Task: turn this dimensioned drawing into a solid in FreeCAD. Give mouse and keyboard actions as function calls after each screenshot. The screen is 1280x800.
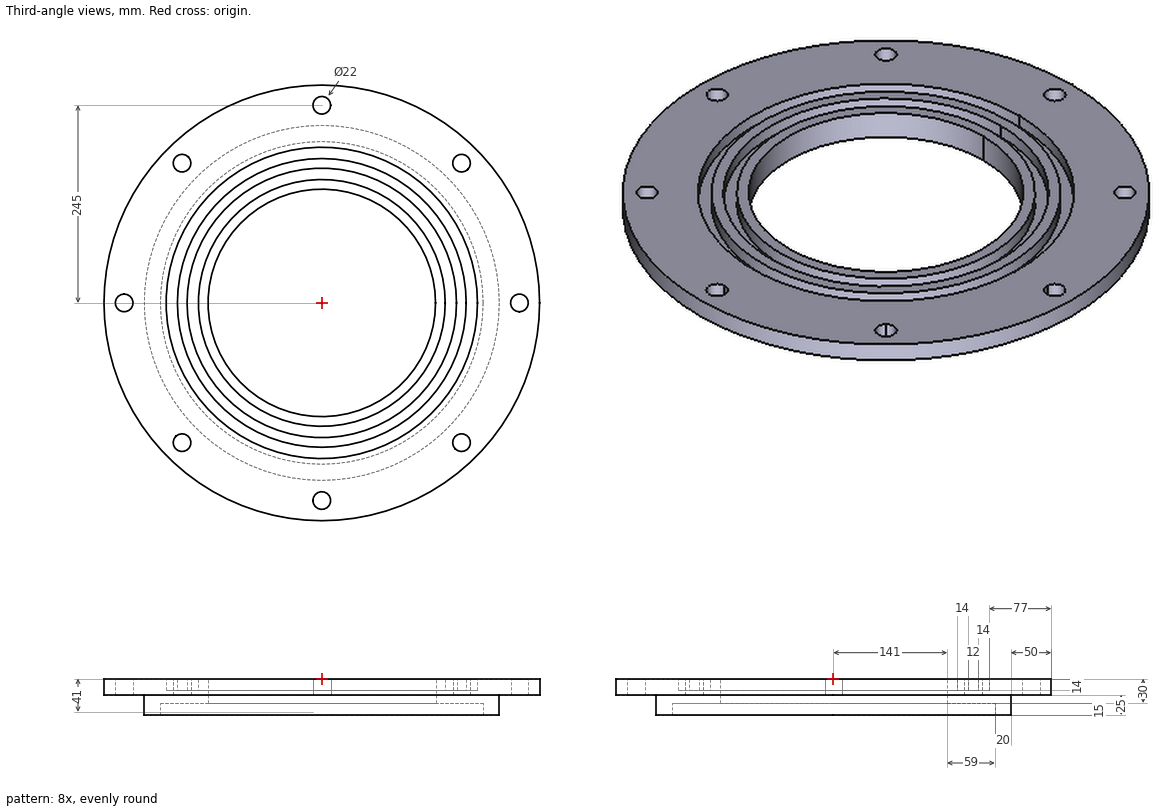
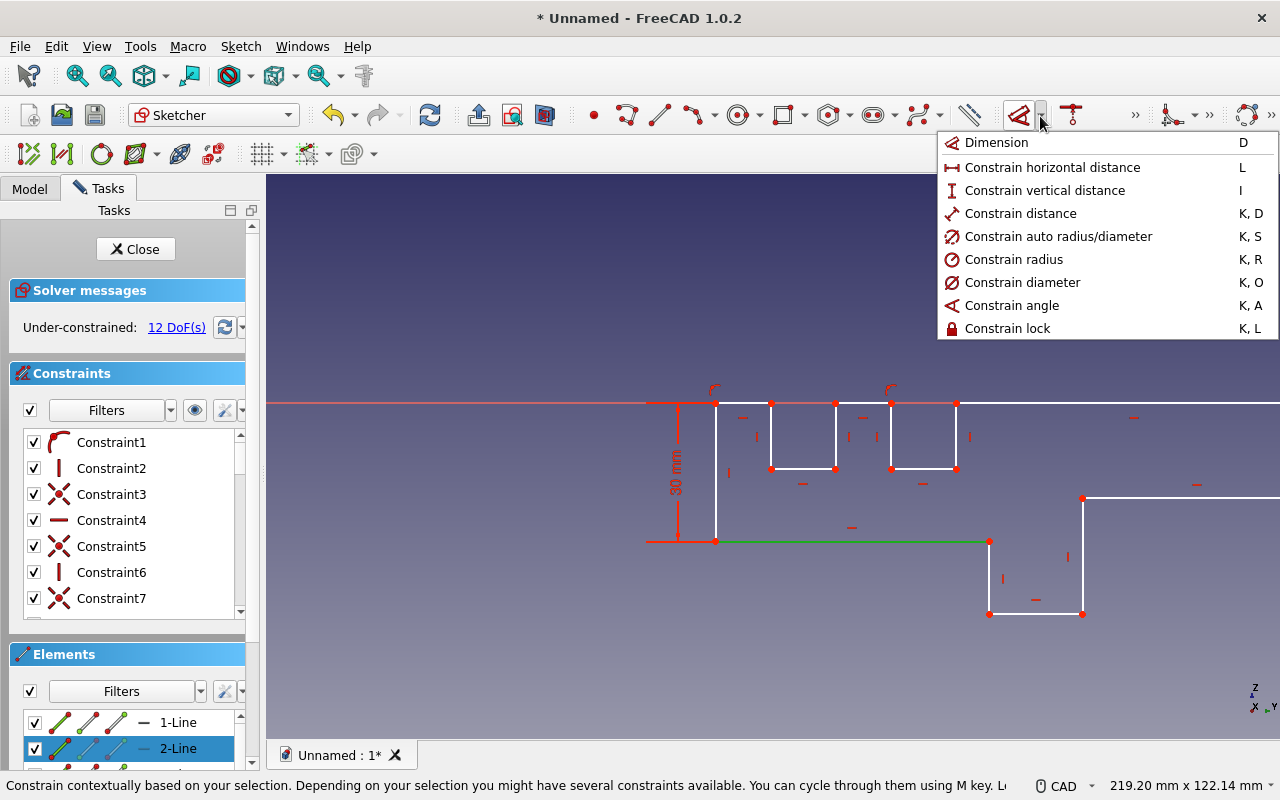
click(1108, 168)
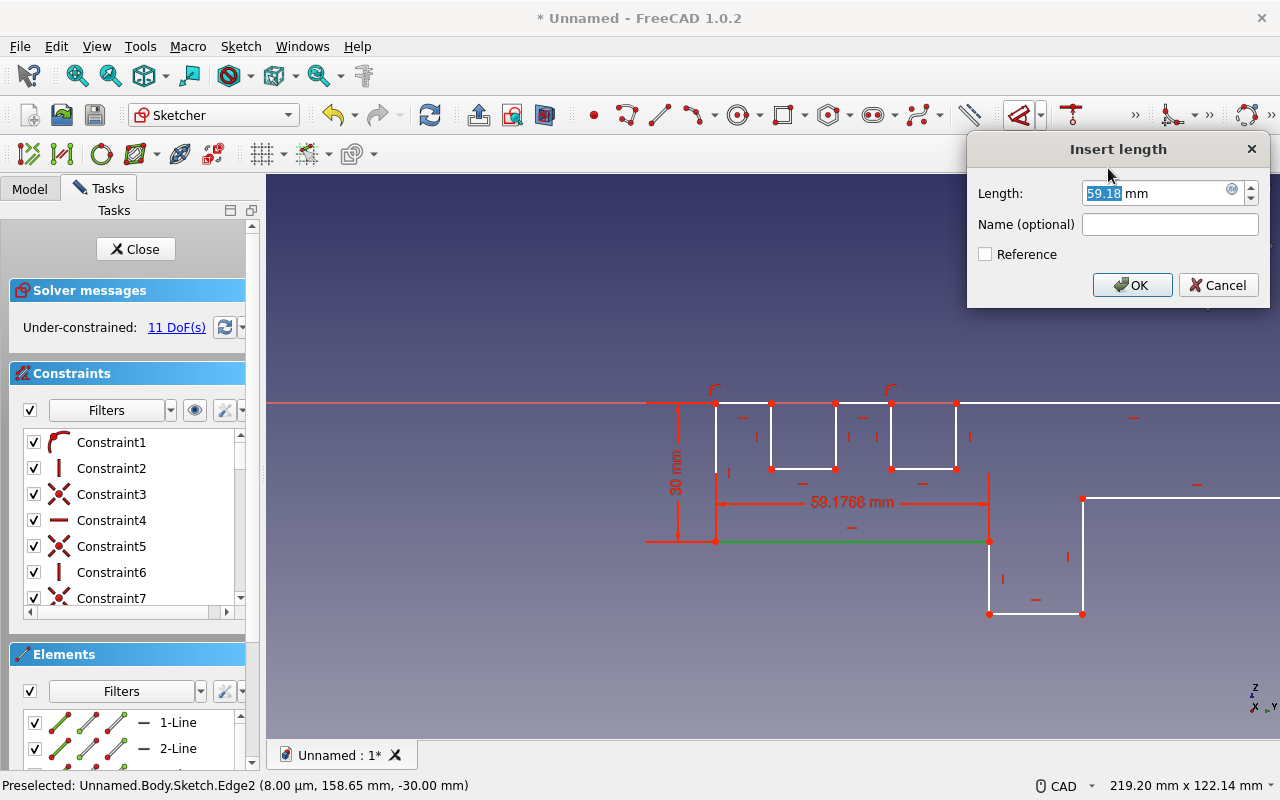
text(59)
key(Return)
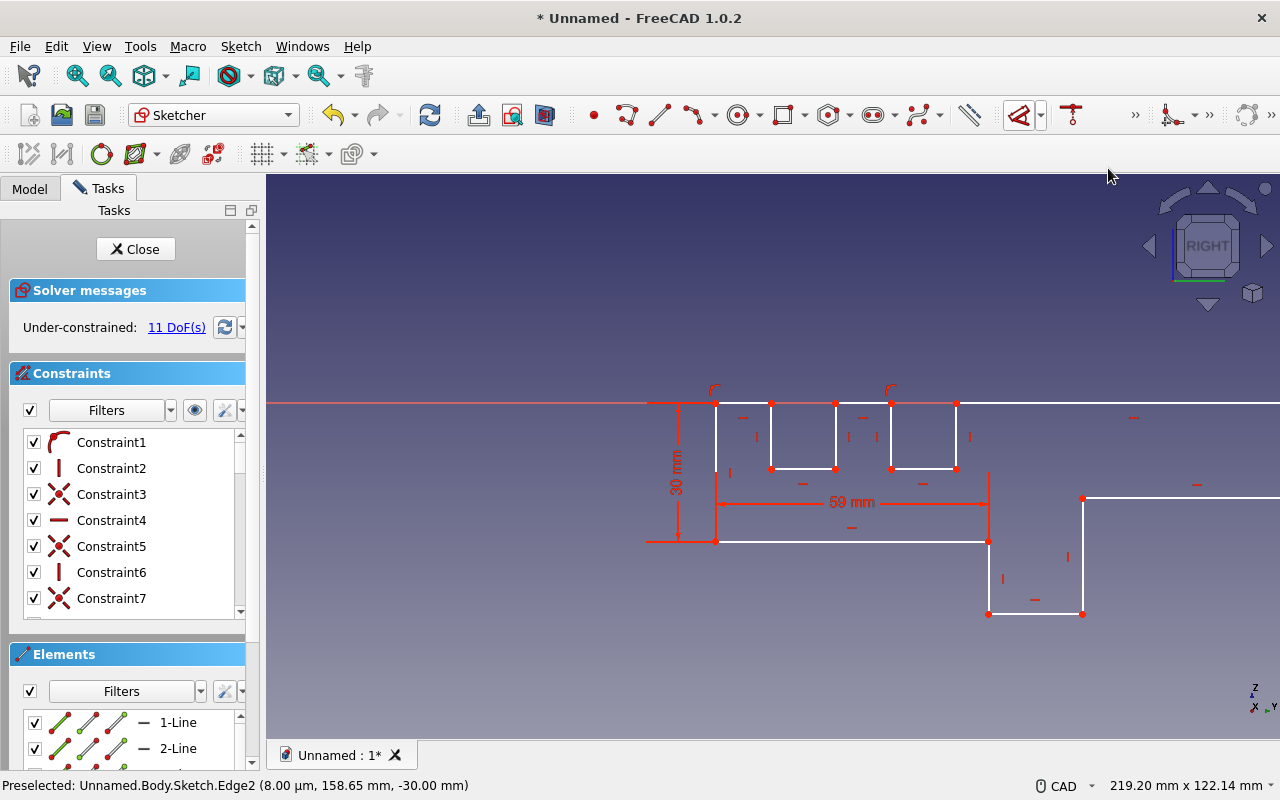
click(989, 564)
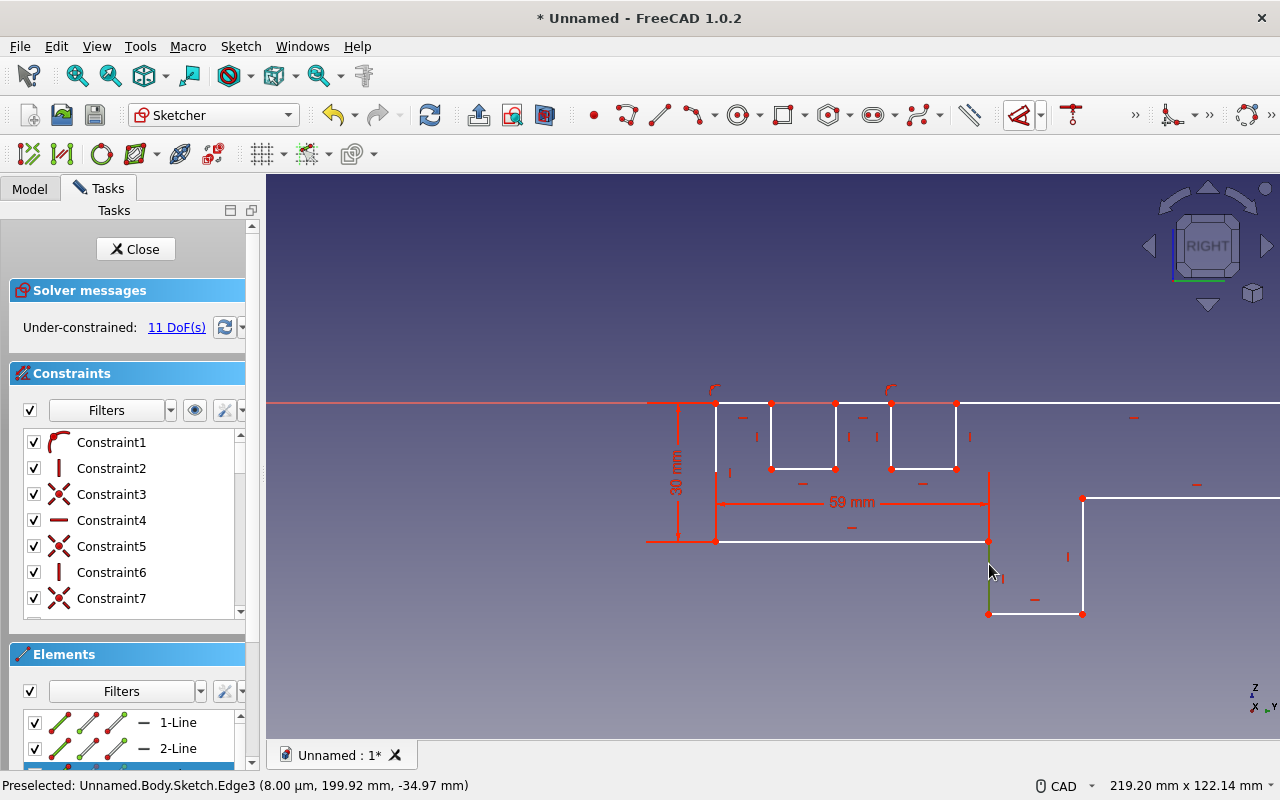
key(i)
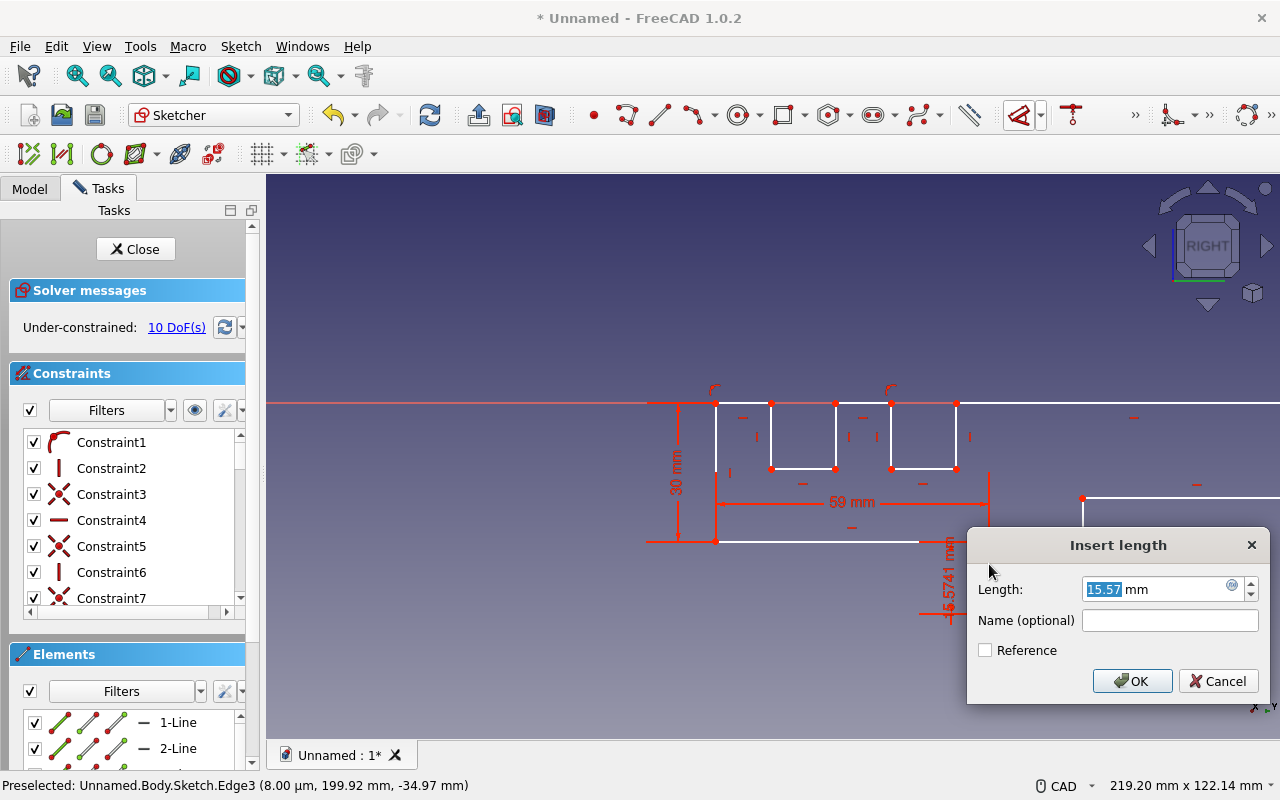
text(15)
key(Return)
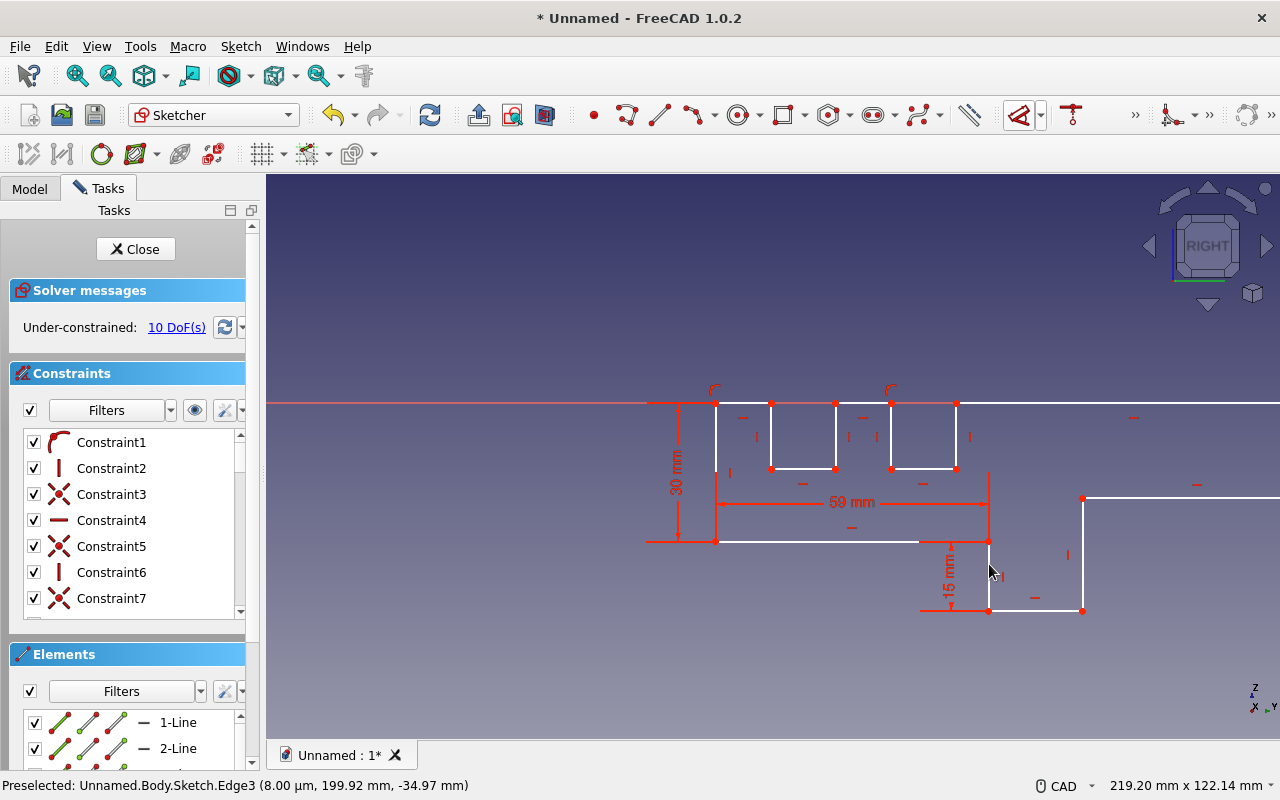
click(1017, 611)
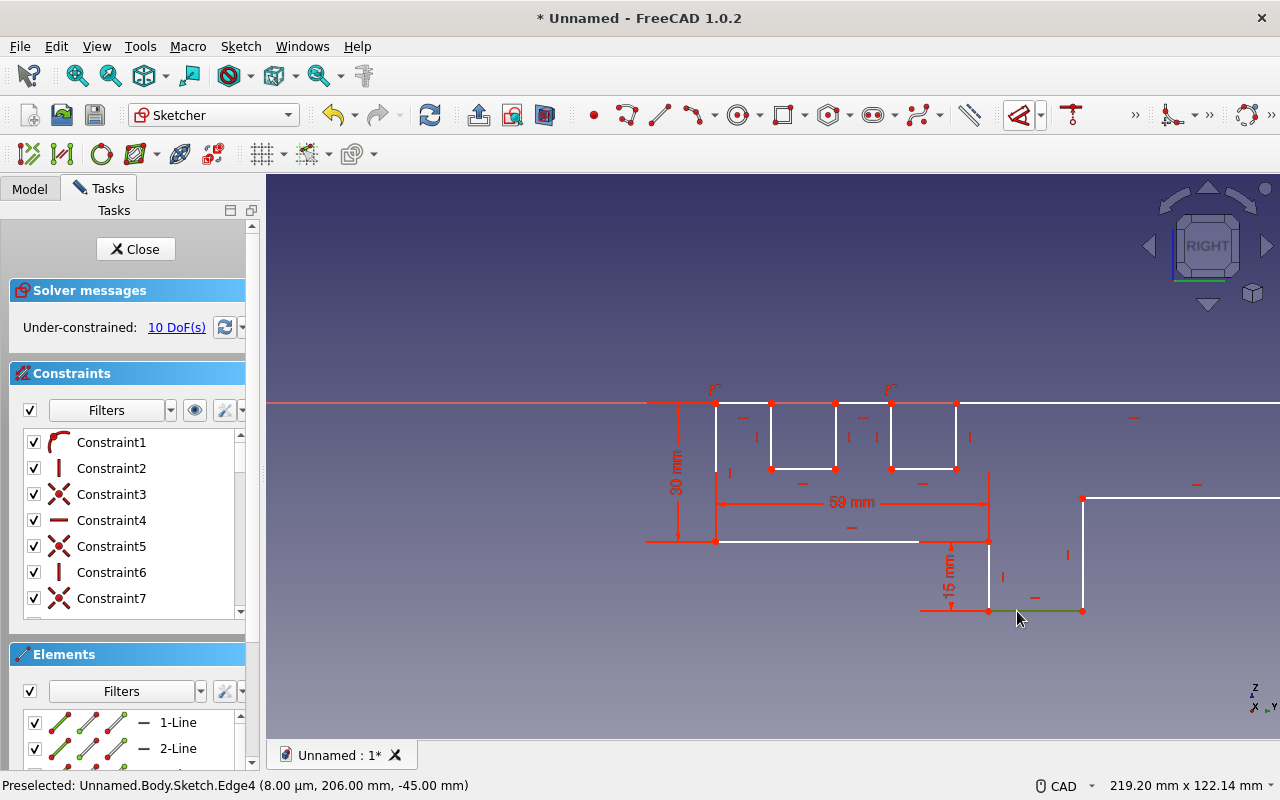
key(l)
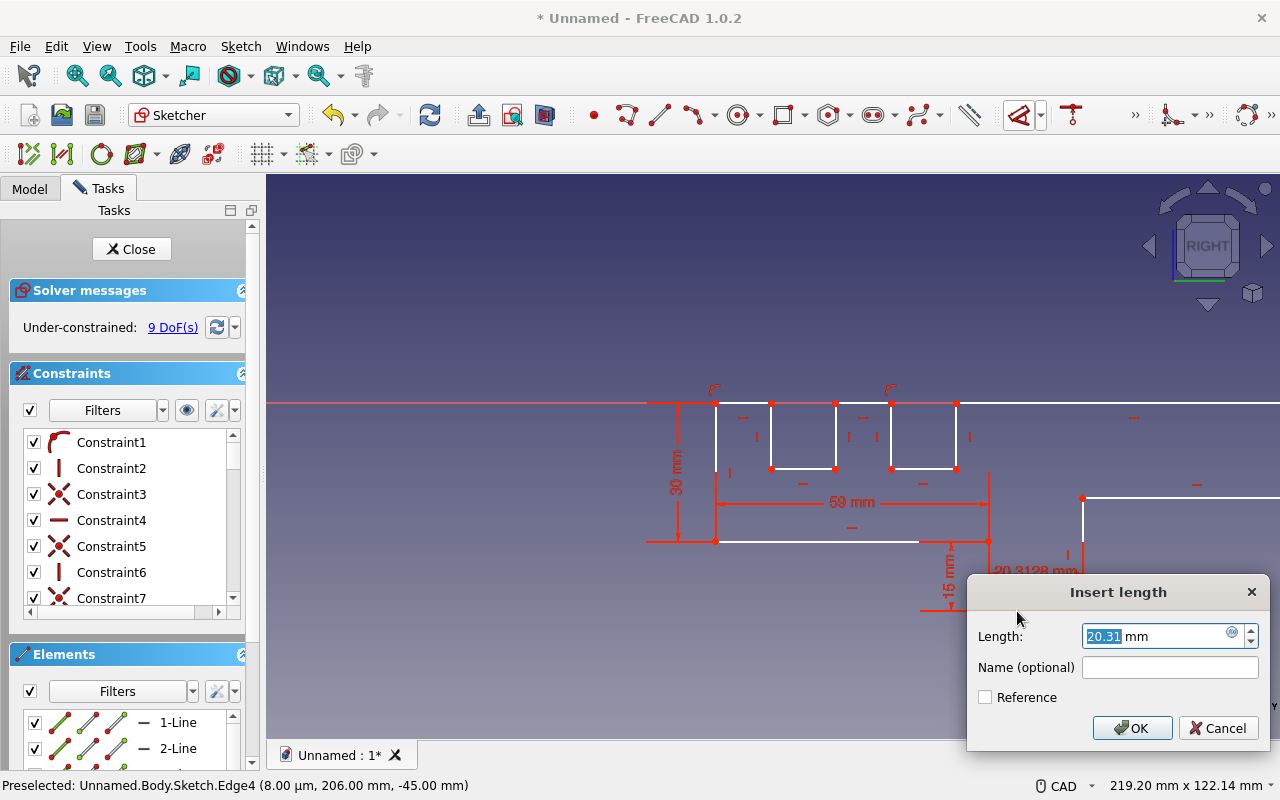
text(20)
key(Return)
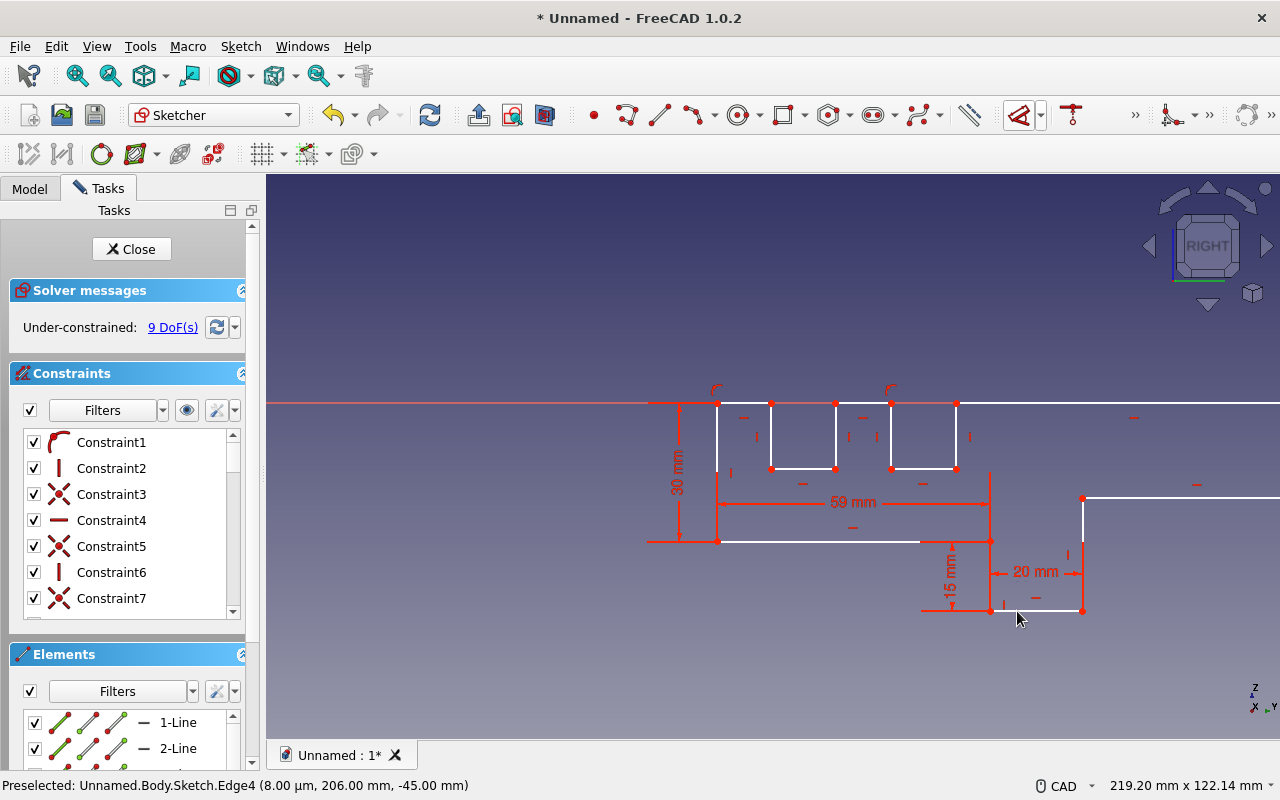
click(1083, 577)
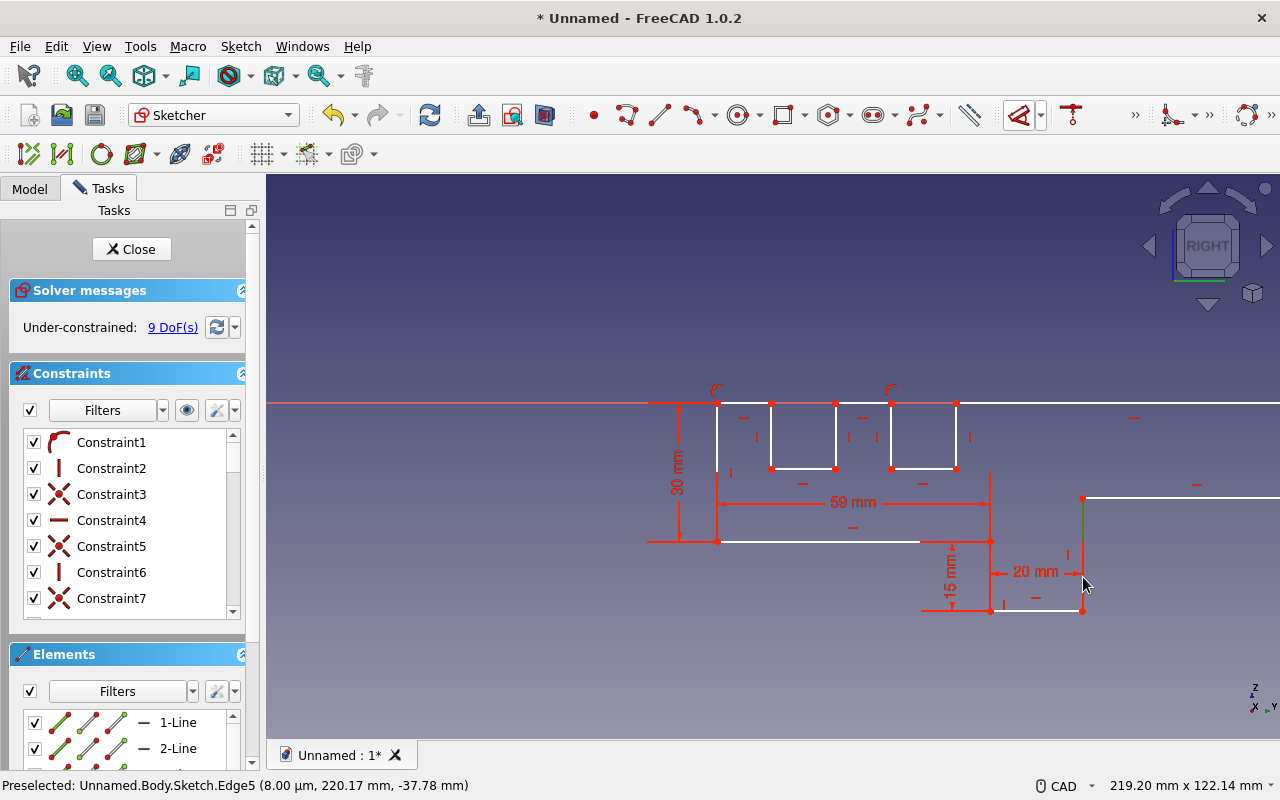
key(i)